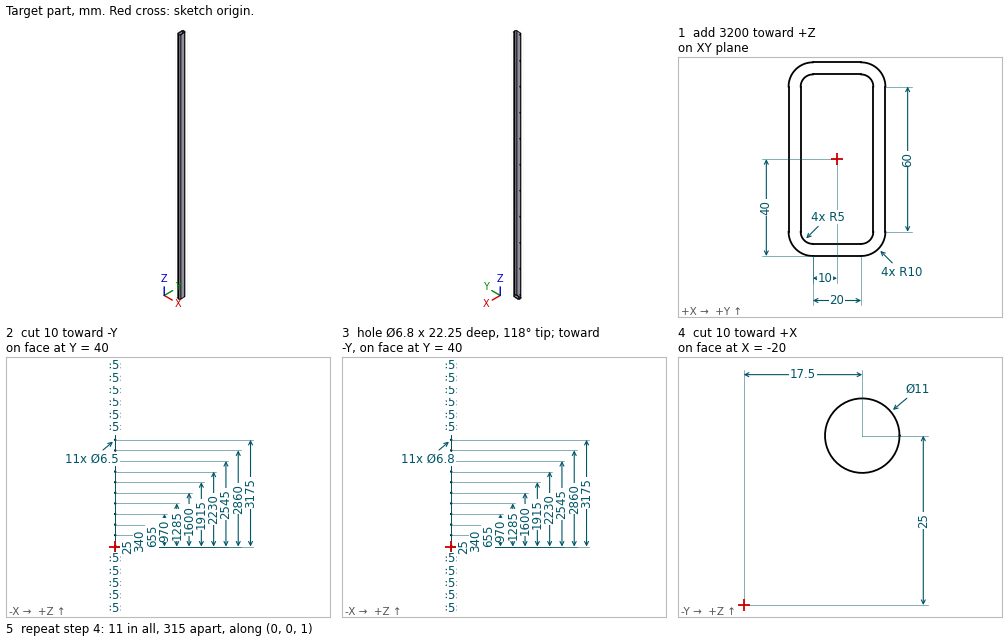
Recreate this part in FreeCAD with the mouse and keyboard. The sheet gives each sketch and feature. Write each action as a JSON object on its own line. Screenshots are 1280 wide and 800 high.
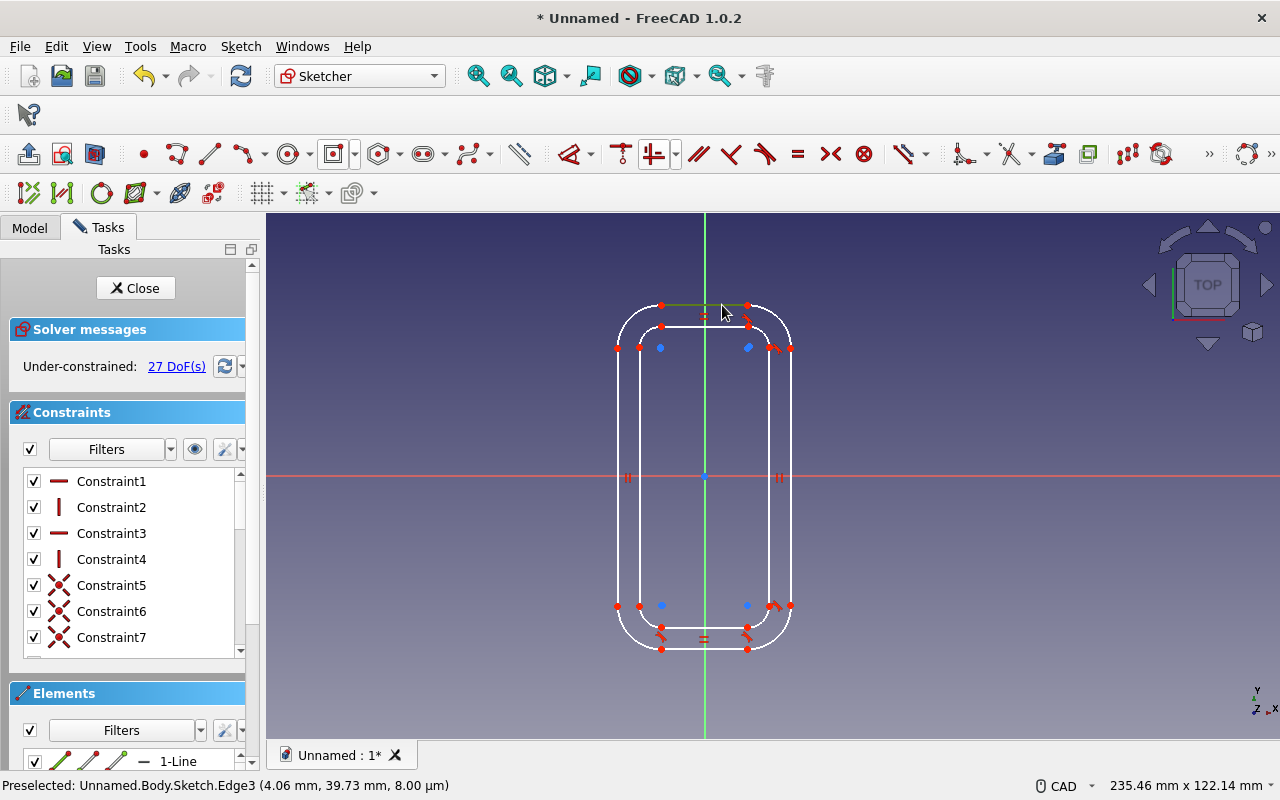
{"action": "left_click", "coordinate": [641, 310]}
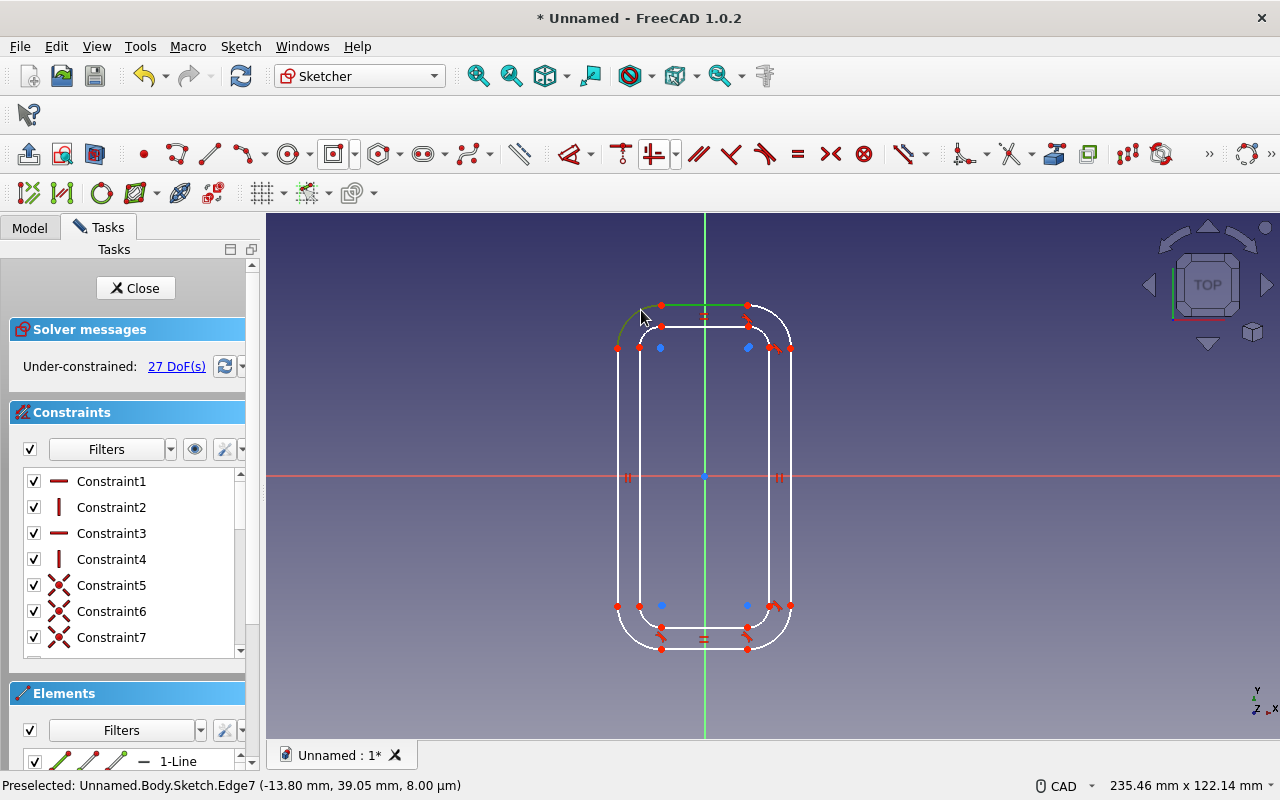
{"action": "left_click", "coordinate": [765, 154]}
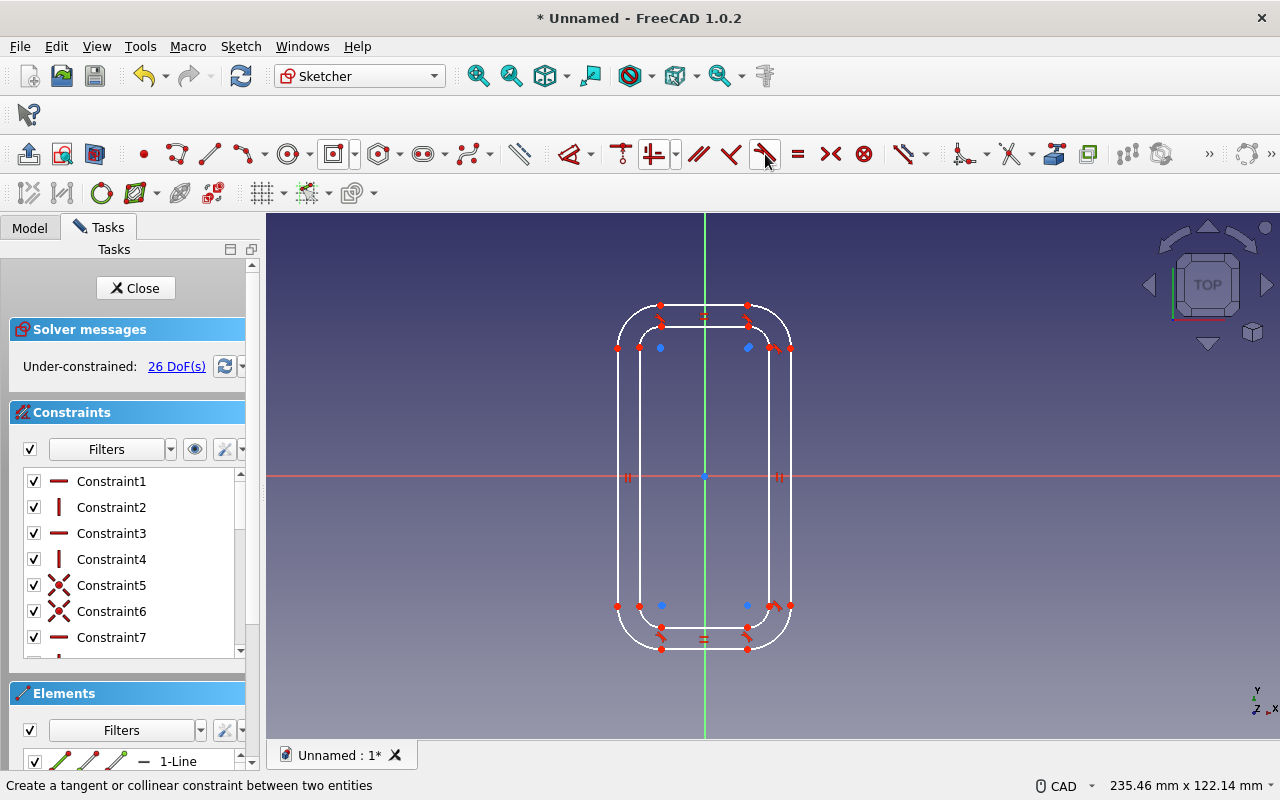
{"action": "left_click", "coordinate": [618, 426]}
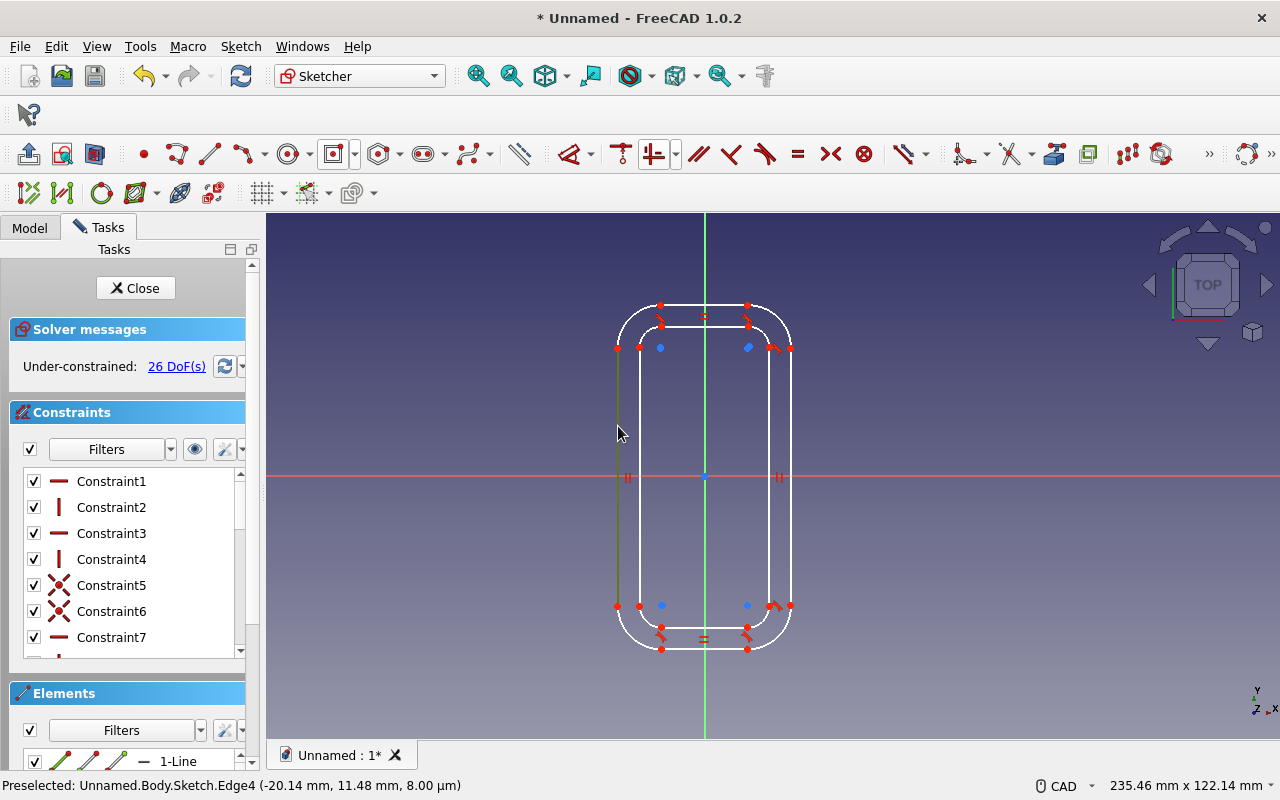
{"action": "left_click", "coordinate": [641, 310]}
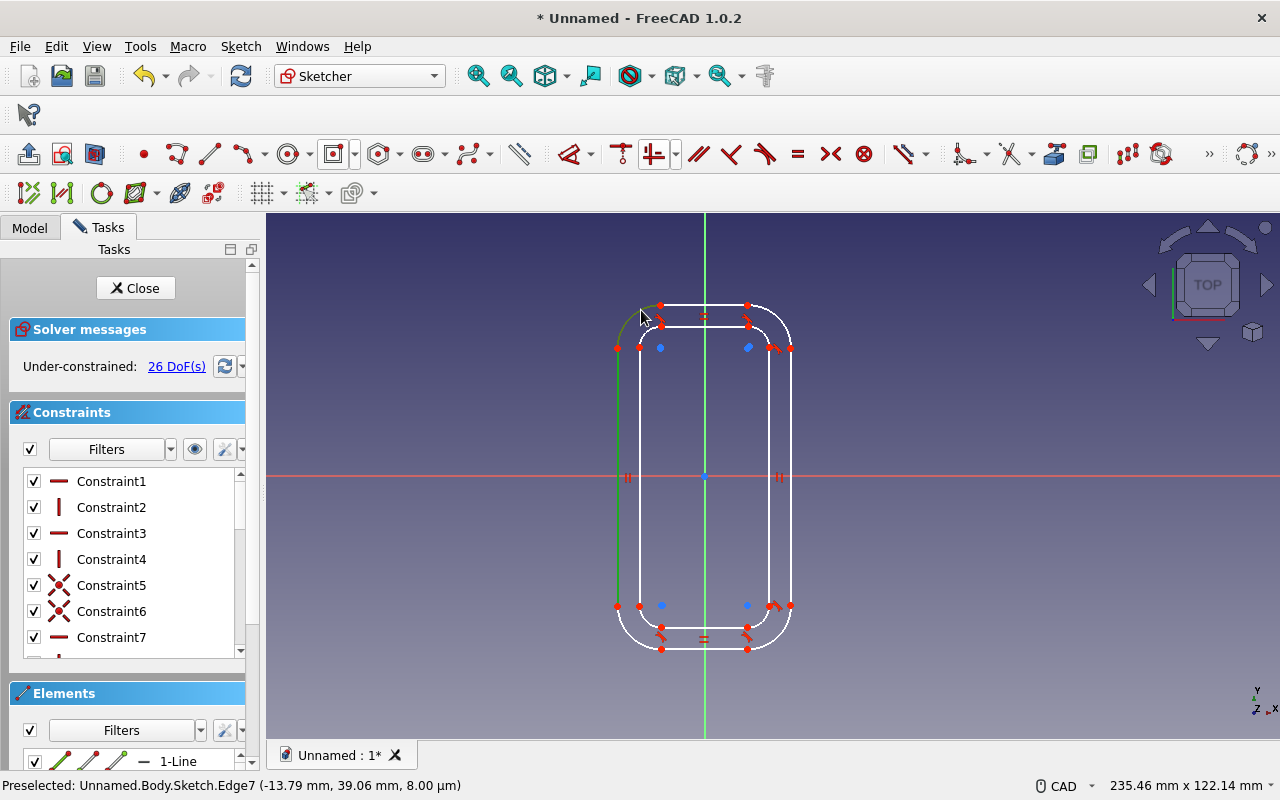
{"action": "key", "text": "t"}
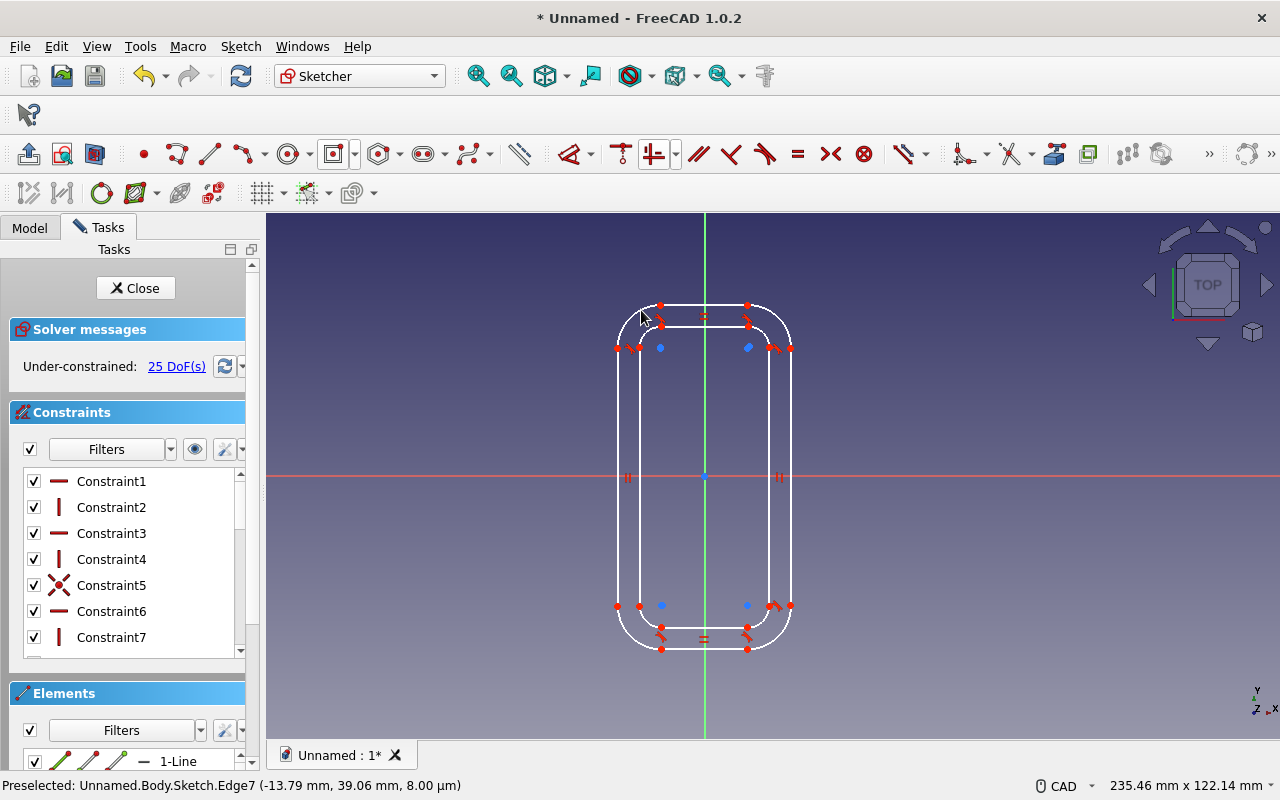
{"action": "left_click", "coordinate": [618, 426]}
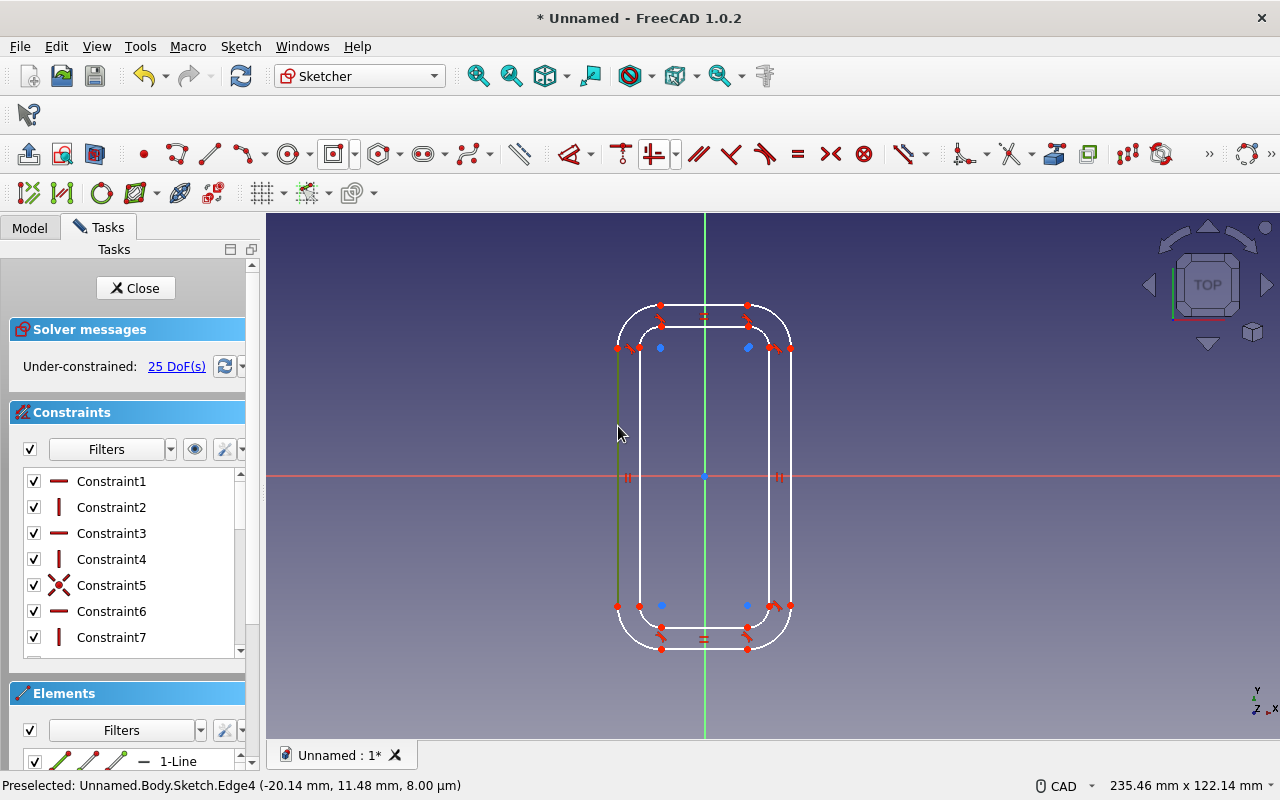
{"action": "left_click", "coordinate": [623, 626]}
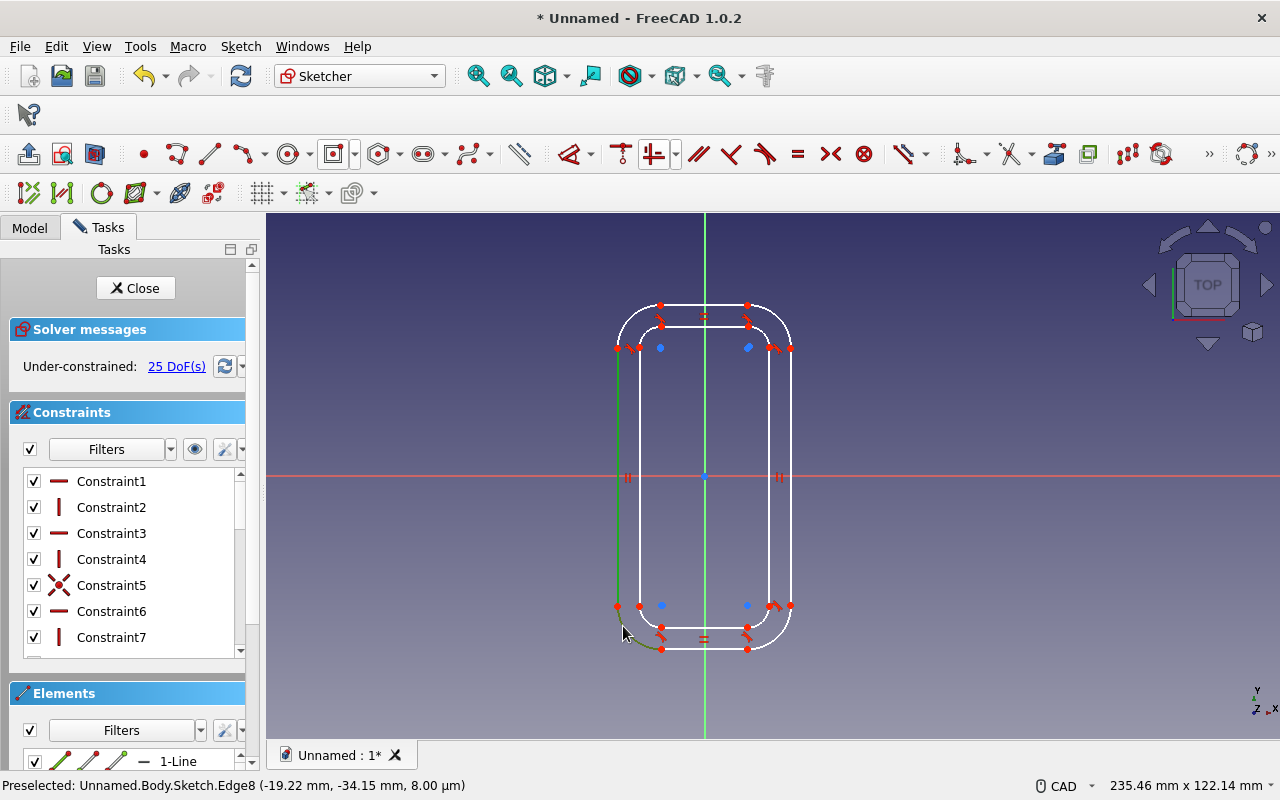
{"action": "left_click", "coordinate": [765, 154]}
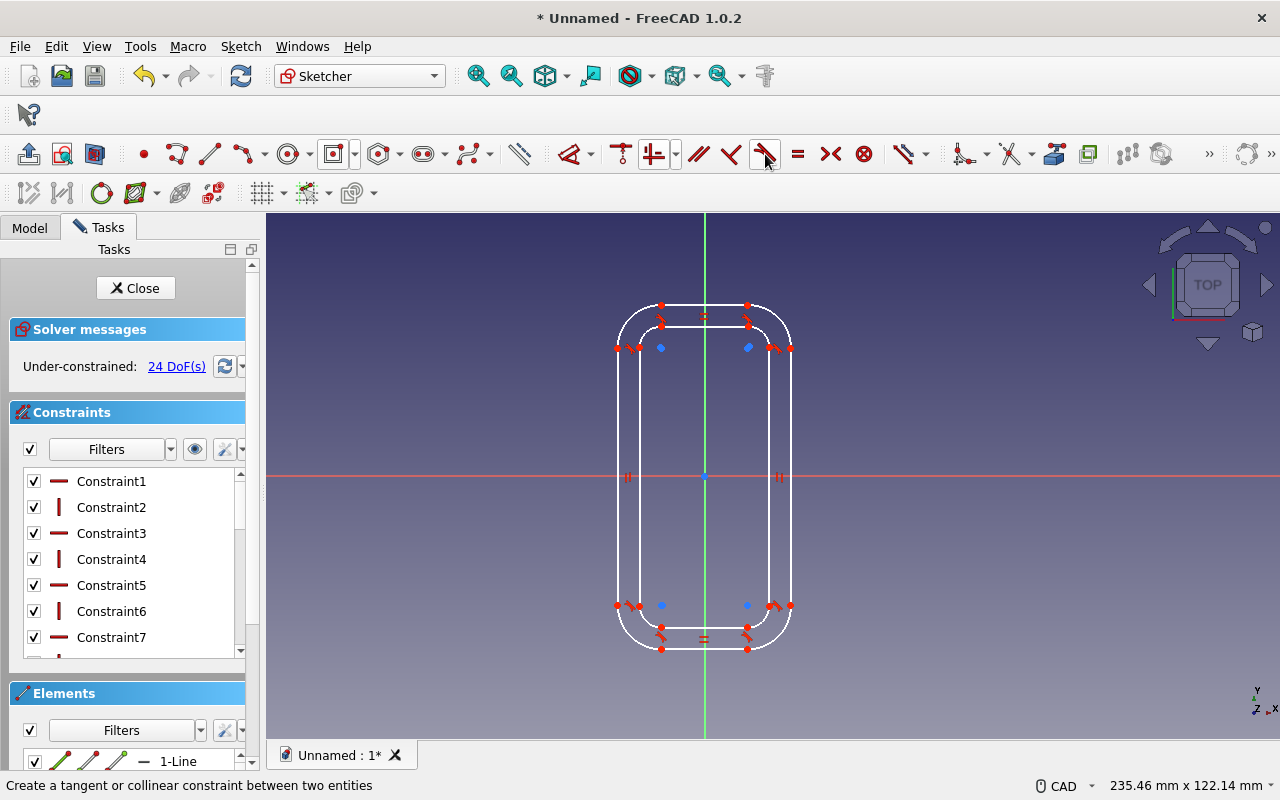
{"action": "left_click", "coordinate": [722, 628]}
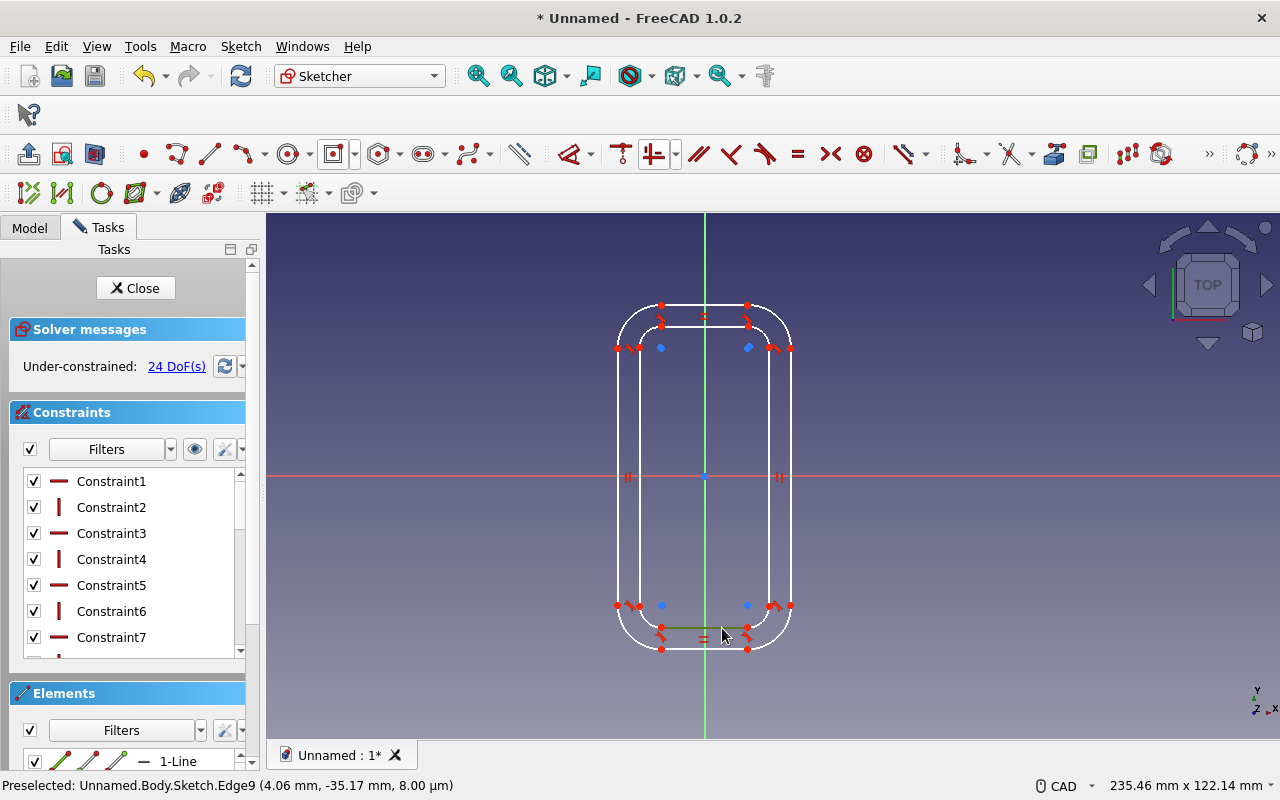
{"action": "scroll", "coordinate": [642, 616], "scroll_direction": "up", "scroll_amount": 2}